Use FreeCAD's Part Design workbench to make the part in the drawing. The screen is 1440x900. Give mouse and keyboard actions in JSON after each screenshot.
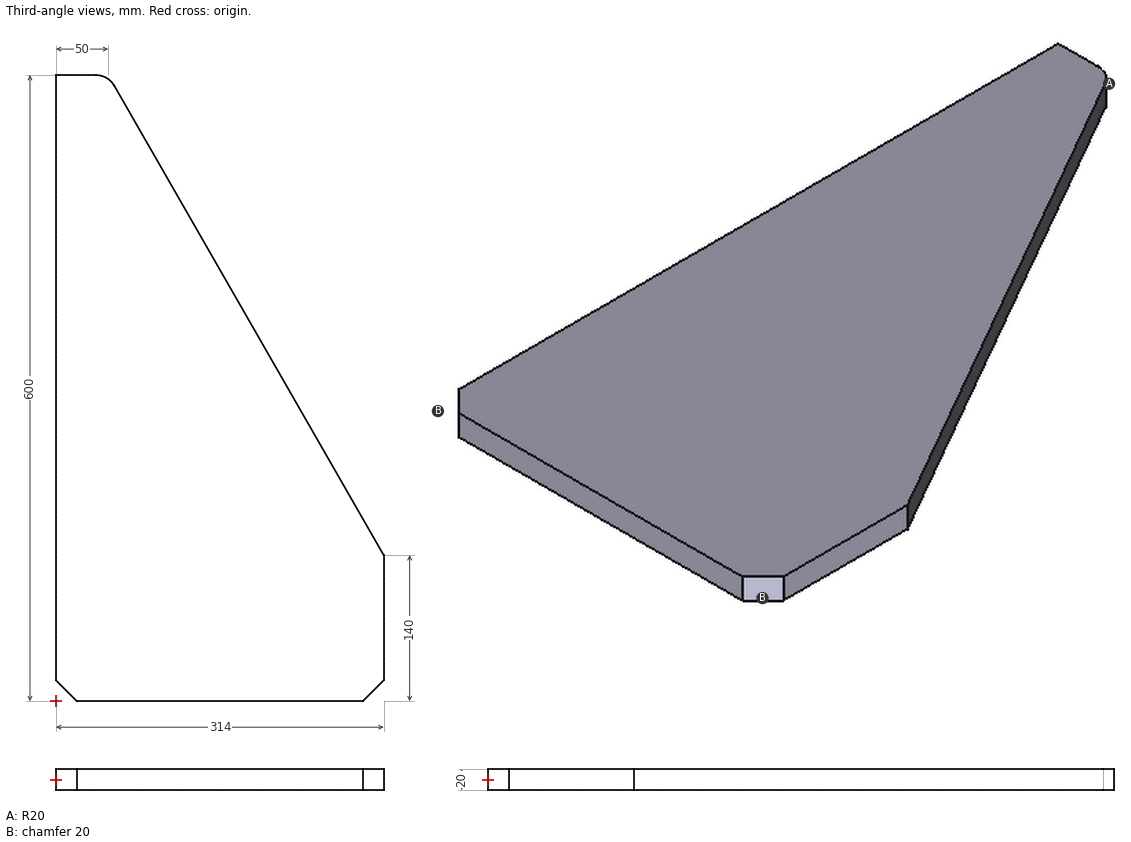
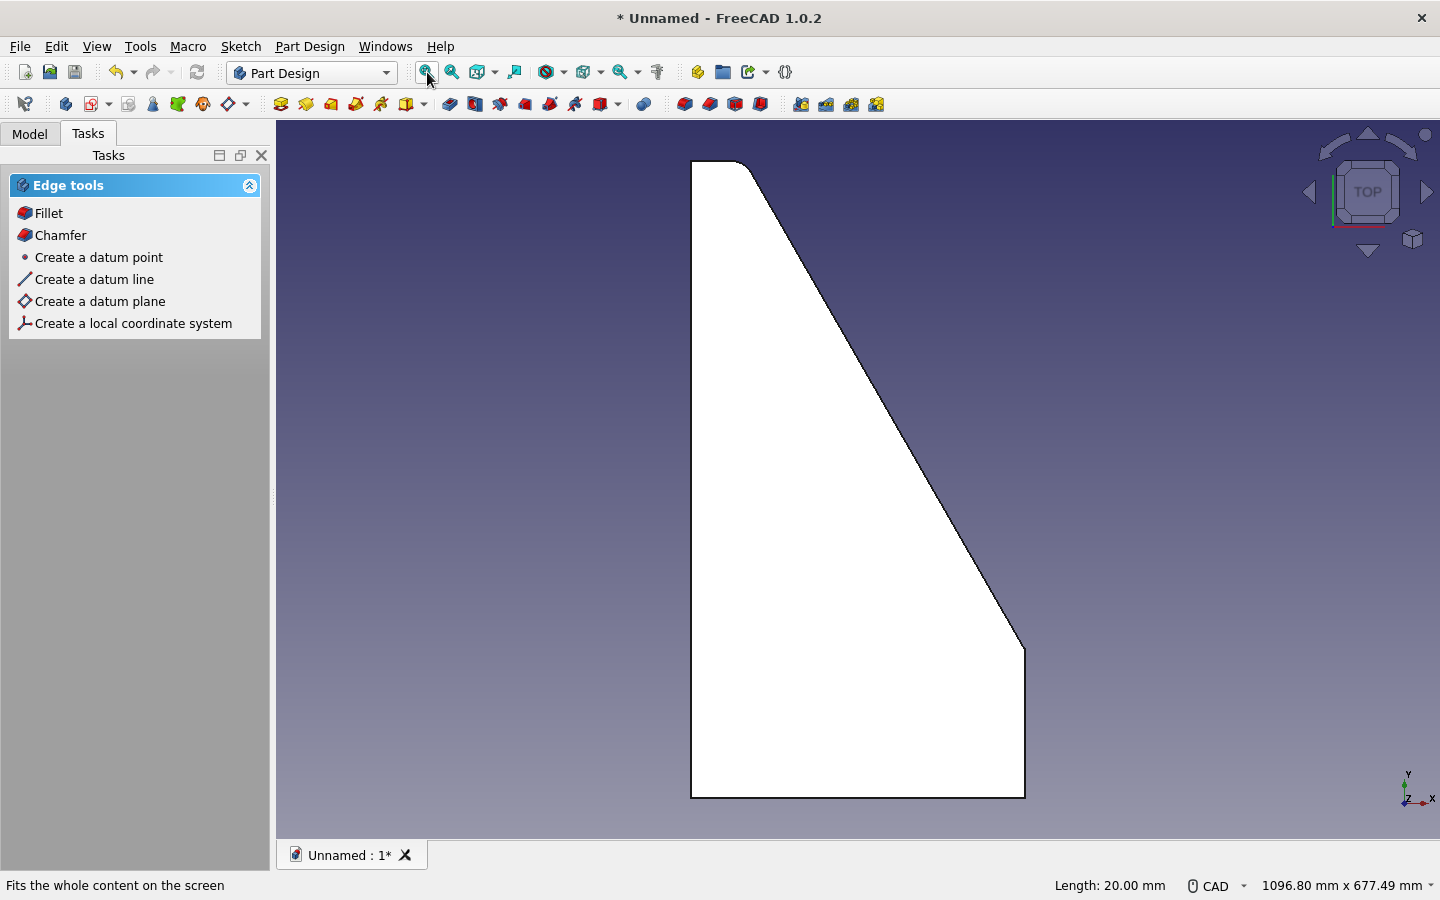
{"action": "key", "text": "1"}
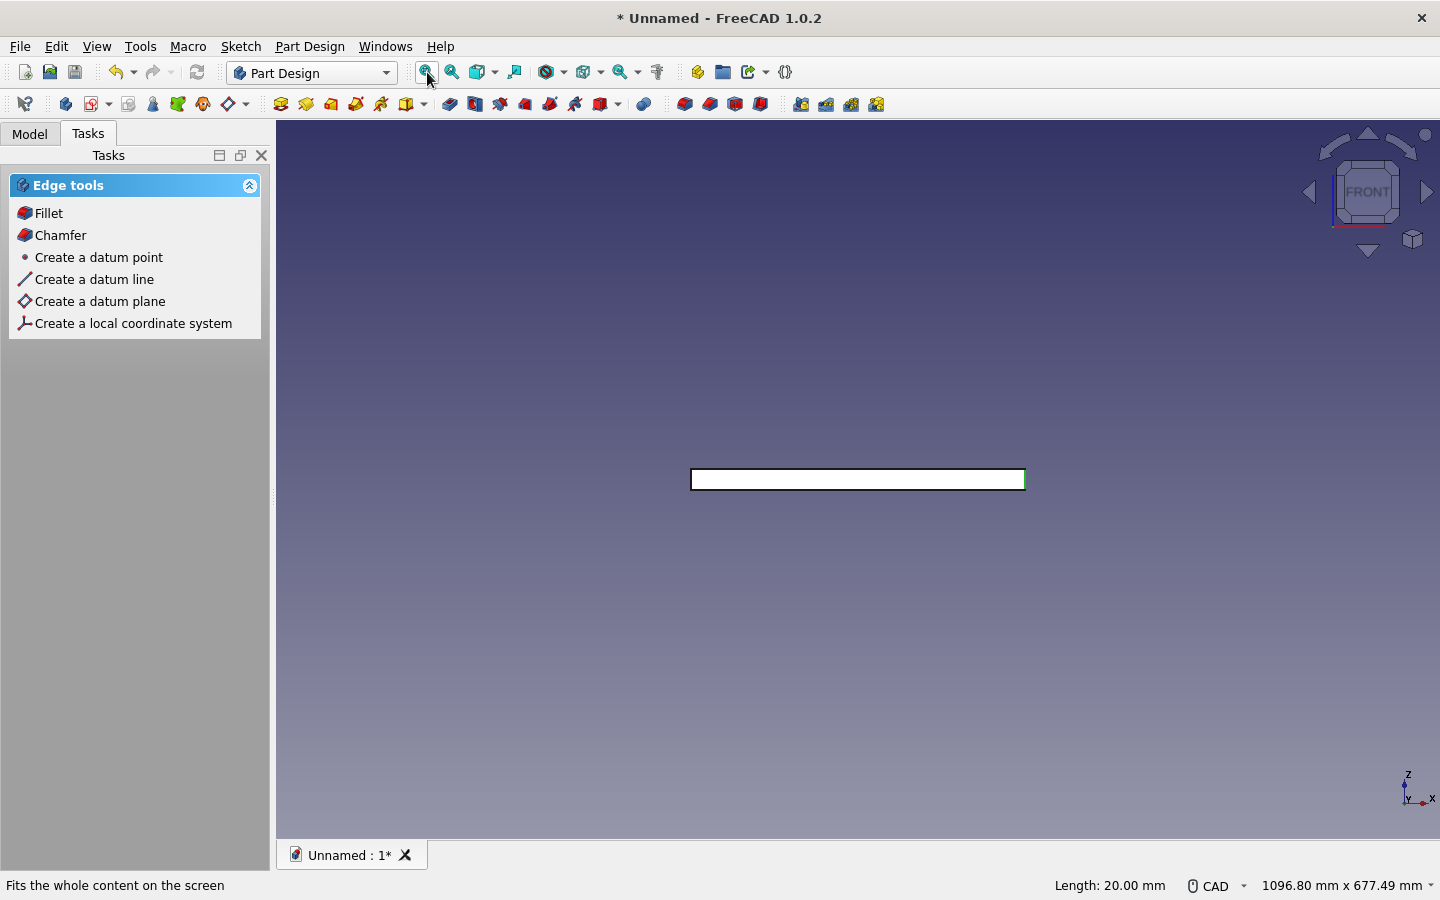
{"action": "key", "text": "v f"}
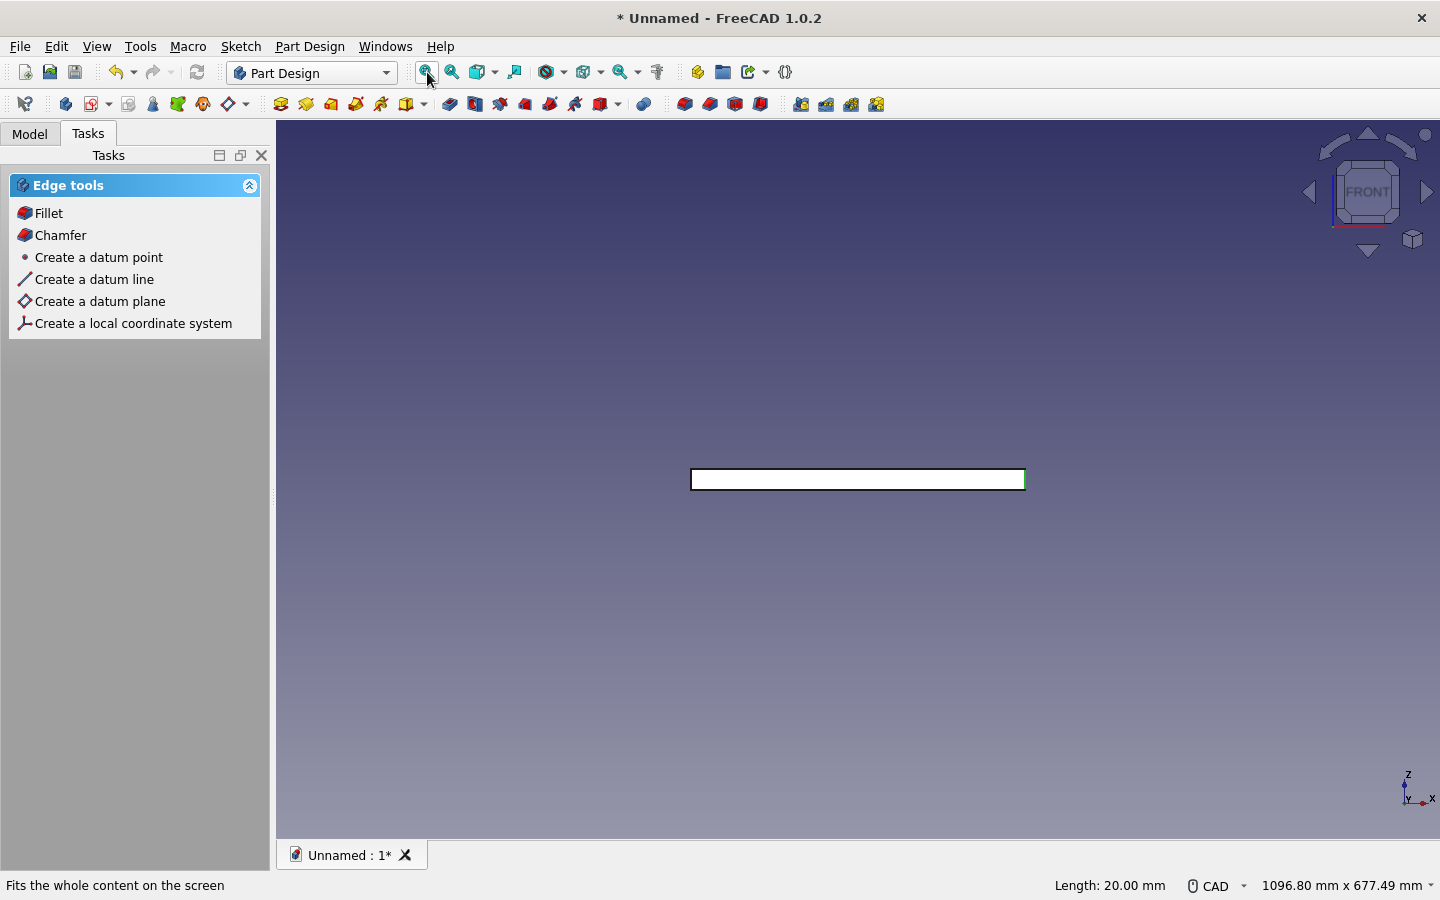
{"action": "left_click", "coordinate": [691, 479], "text": "ctrl"}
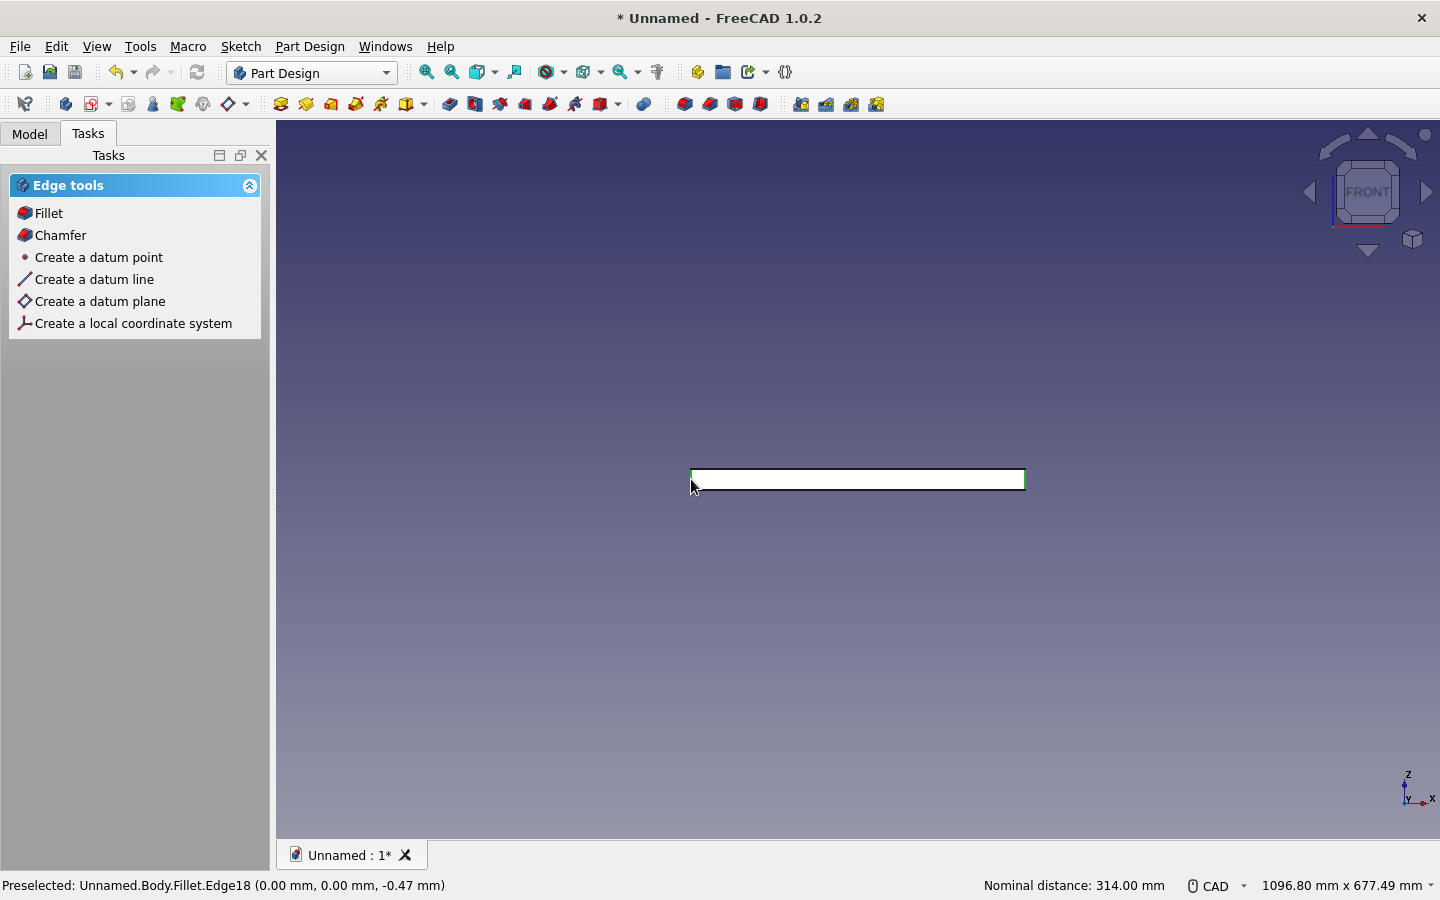
{"action": "left_click", "coordinate": [710, 104]}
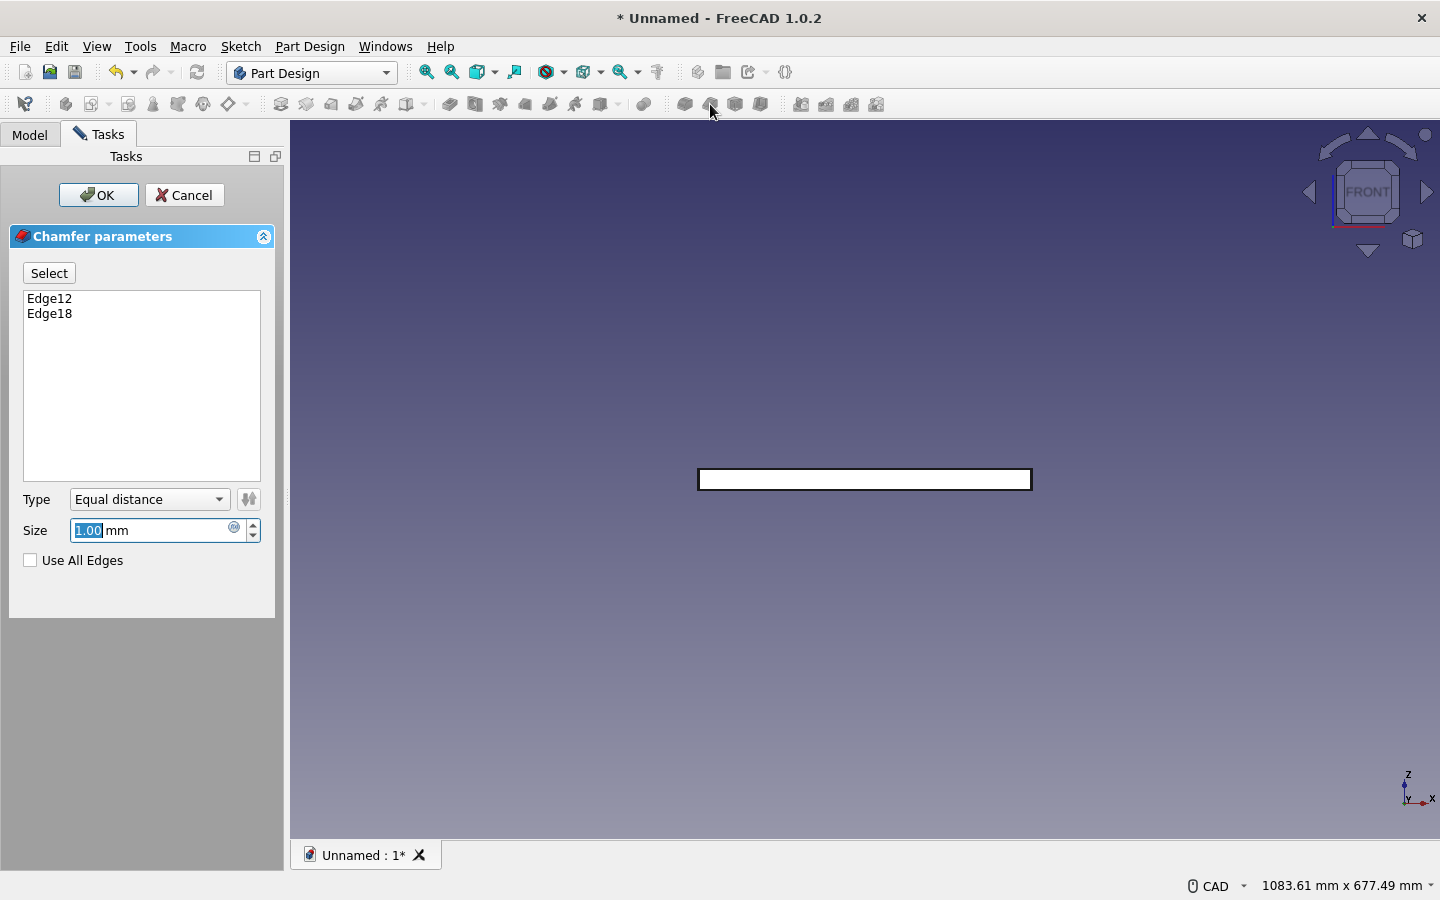
{"action": "type", "text": "20"}
{"action": "key", "text": "Tab"}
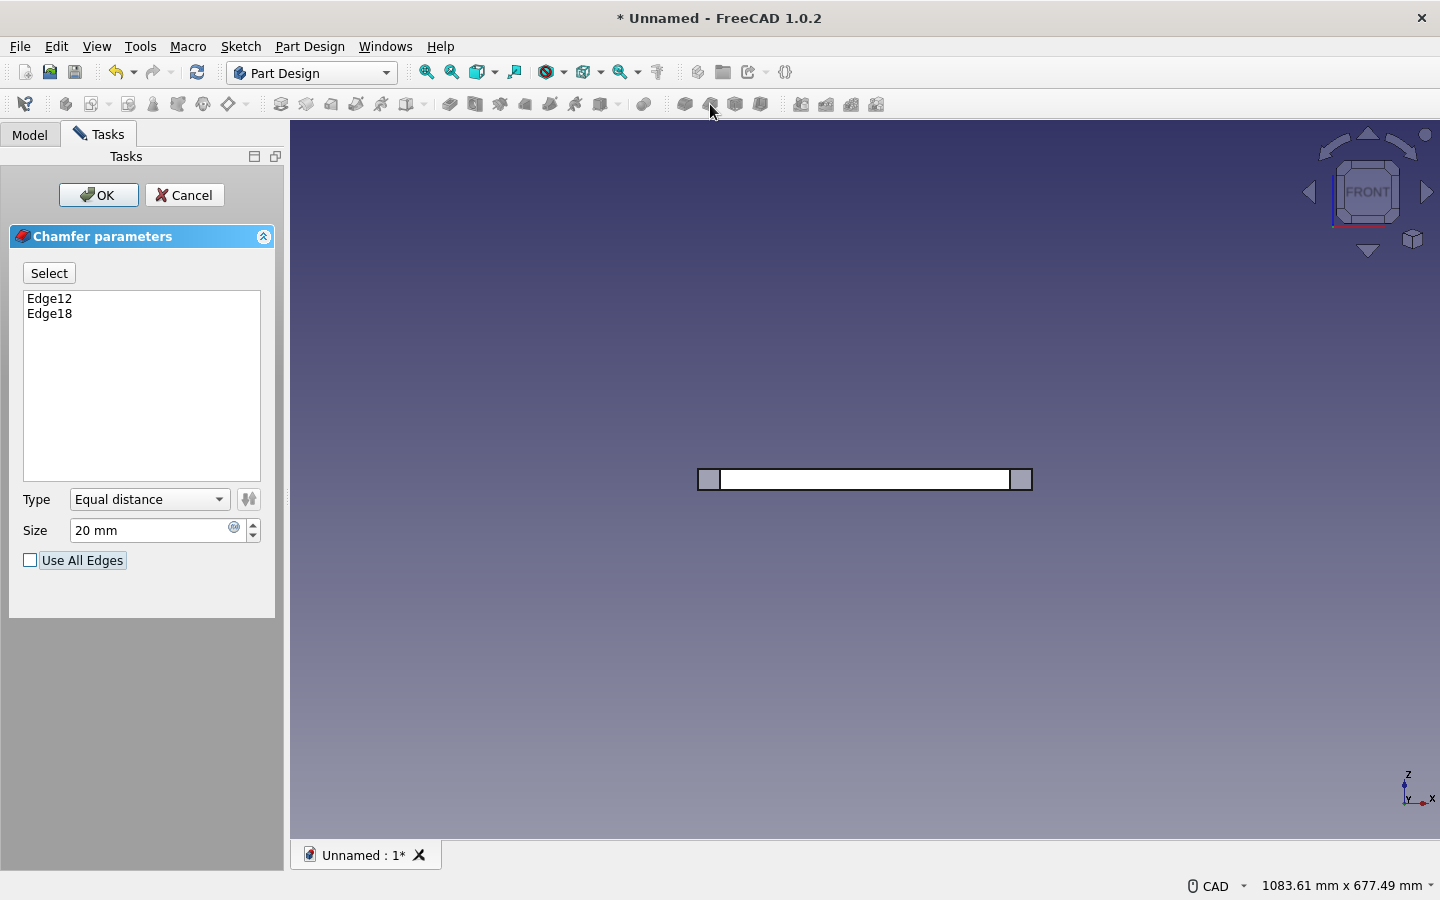
{"action": "left_click", "coordinate": [99, 195]}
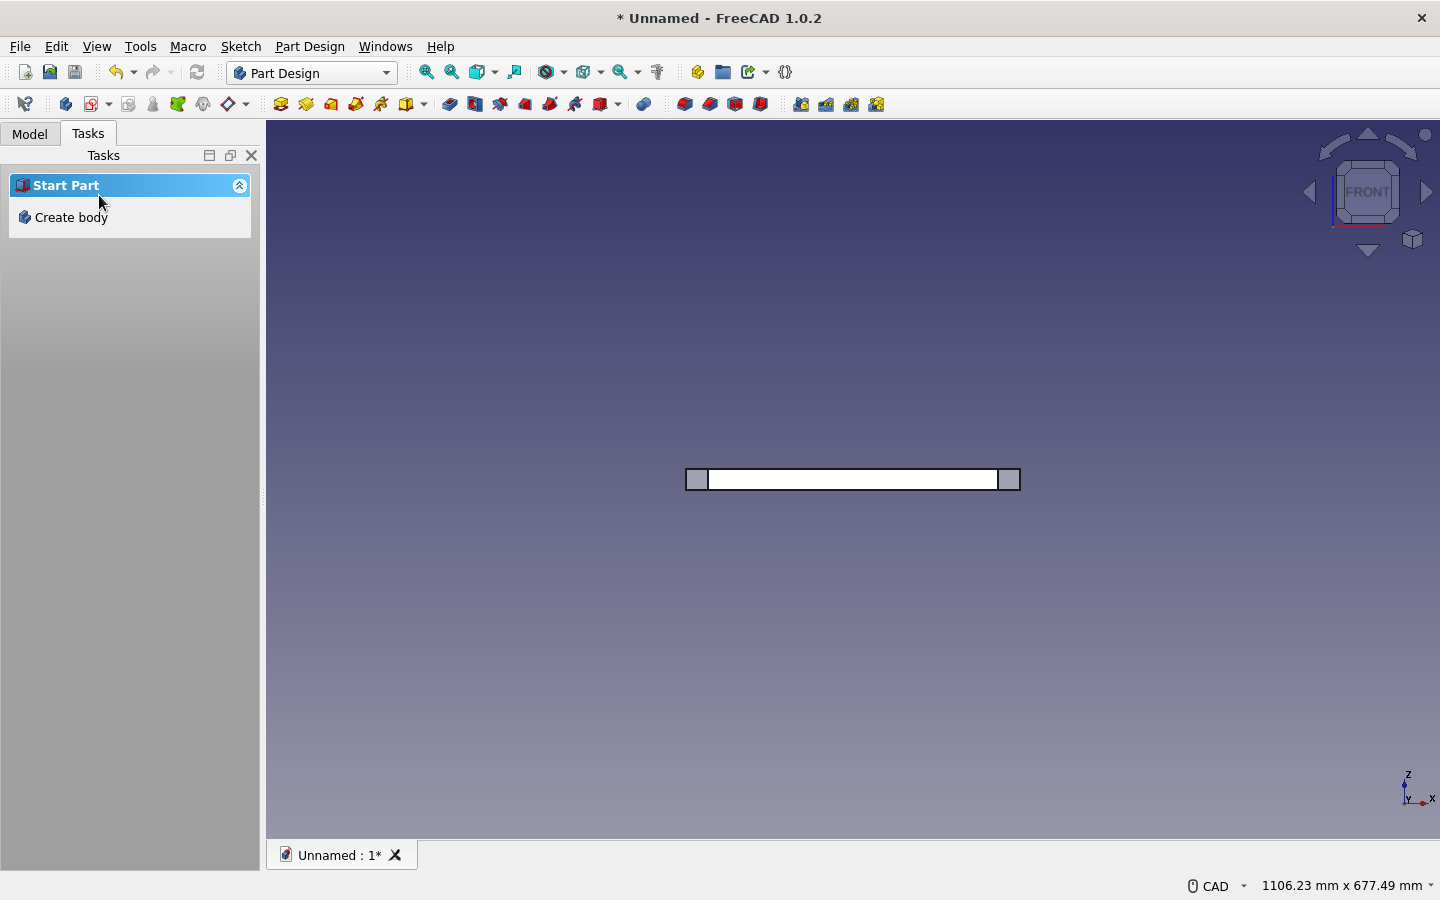
{"action": "key", "text": "0"}